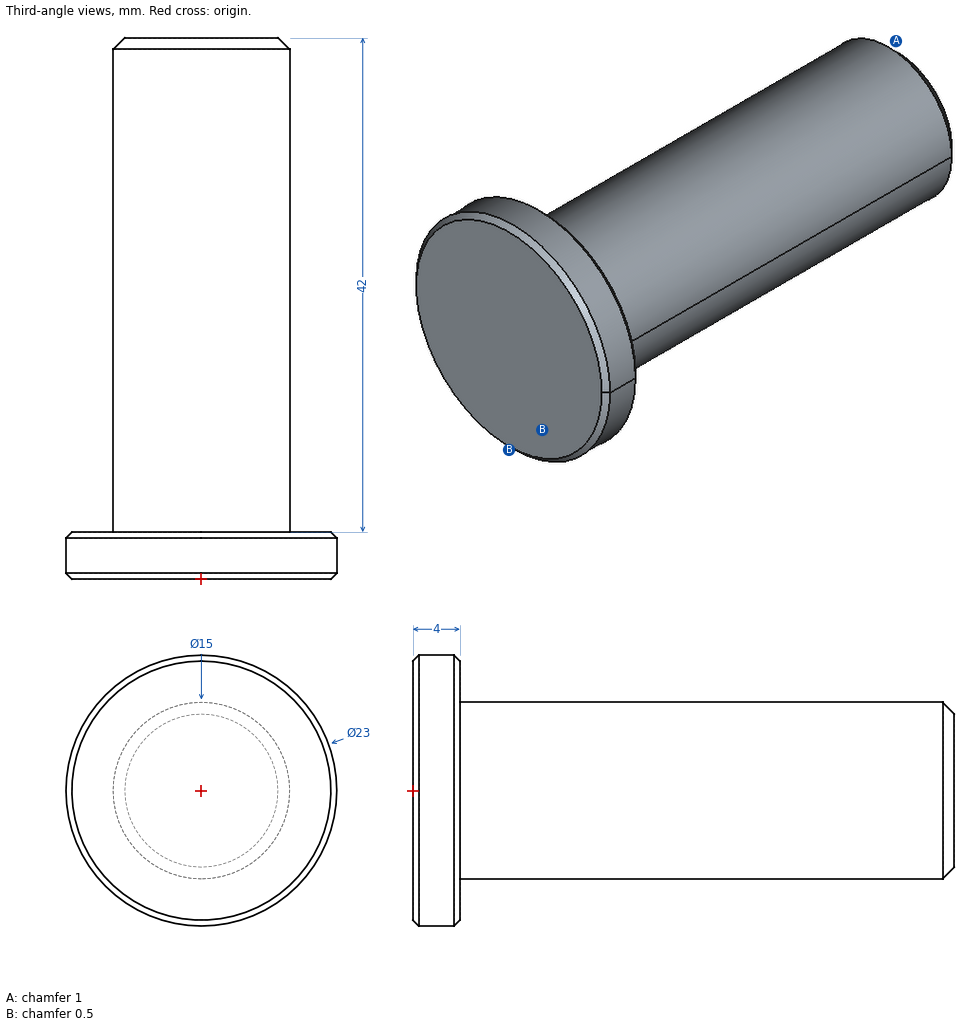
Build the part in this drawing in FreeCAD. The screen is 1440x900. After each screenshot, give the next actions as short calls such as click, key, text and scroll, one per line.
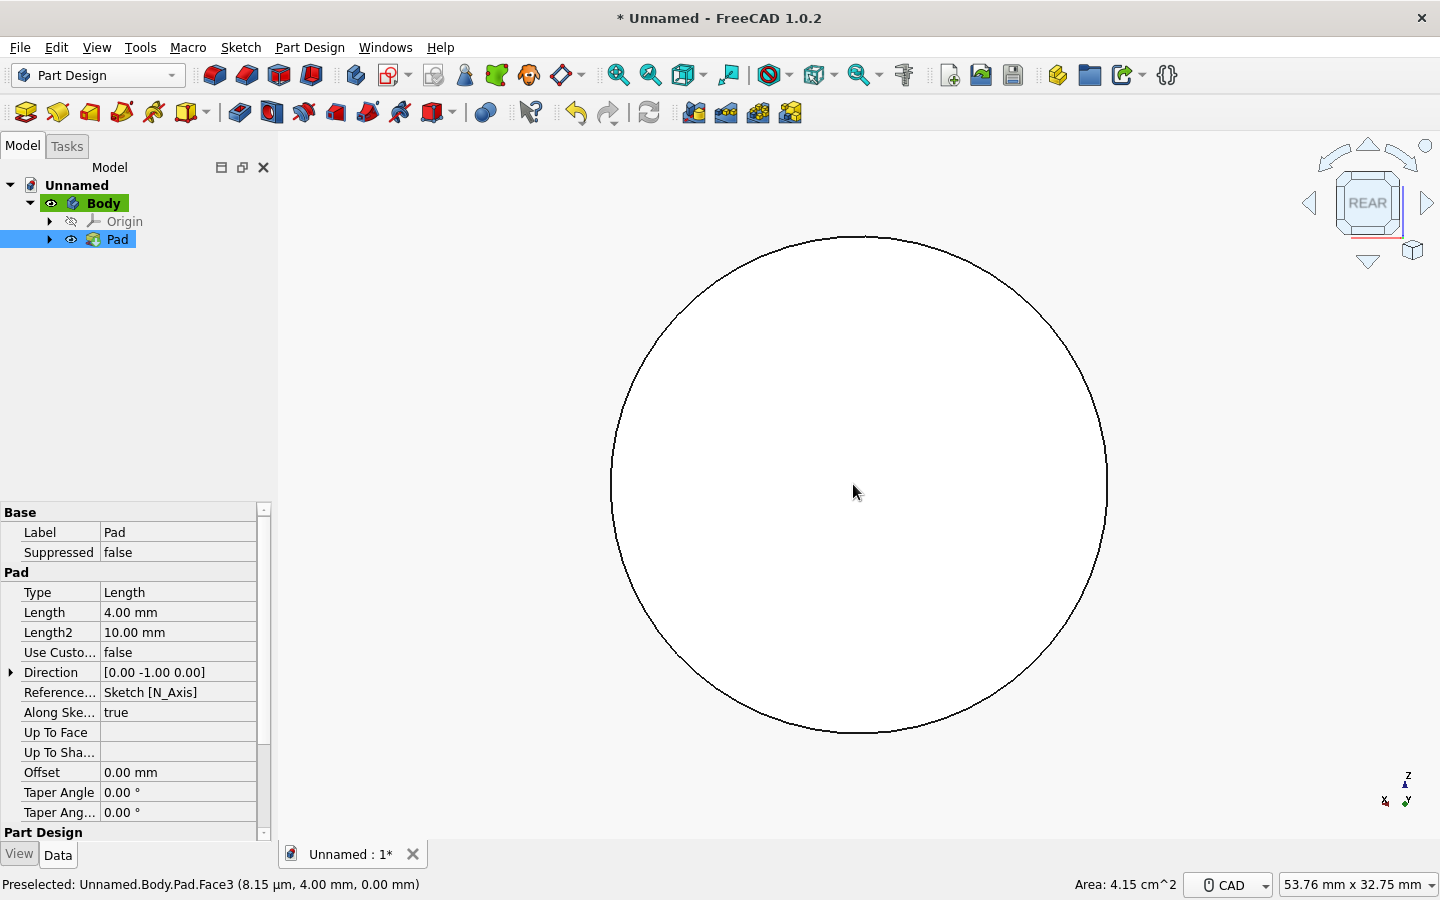
click(388, 76)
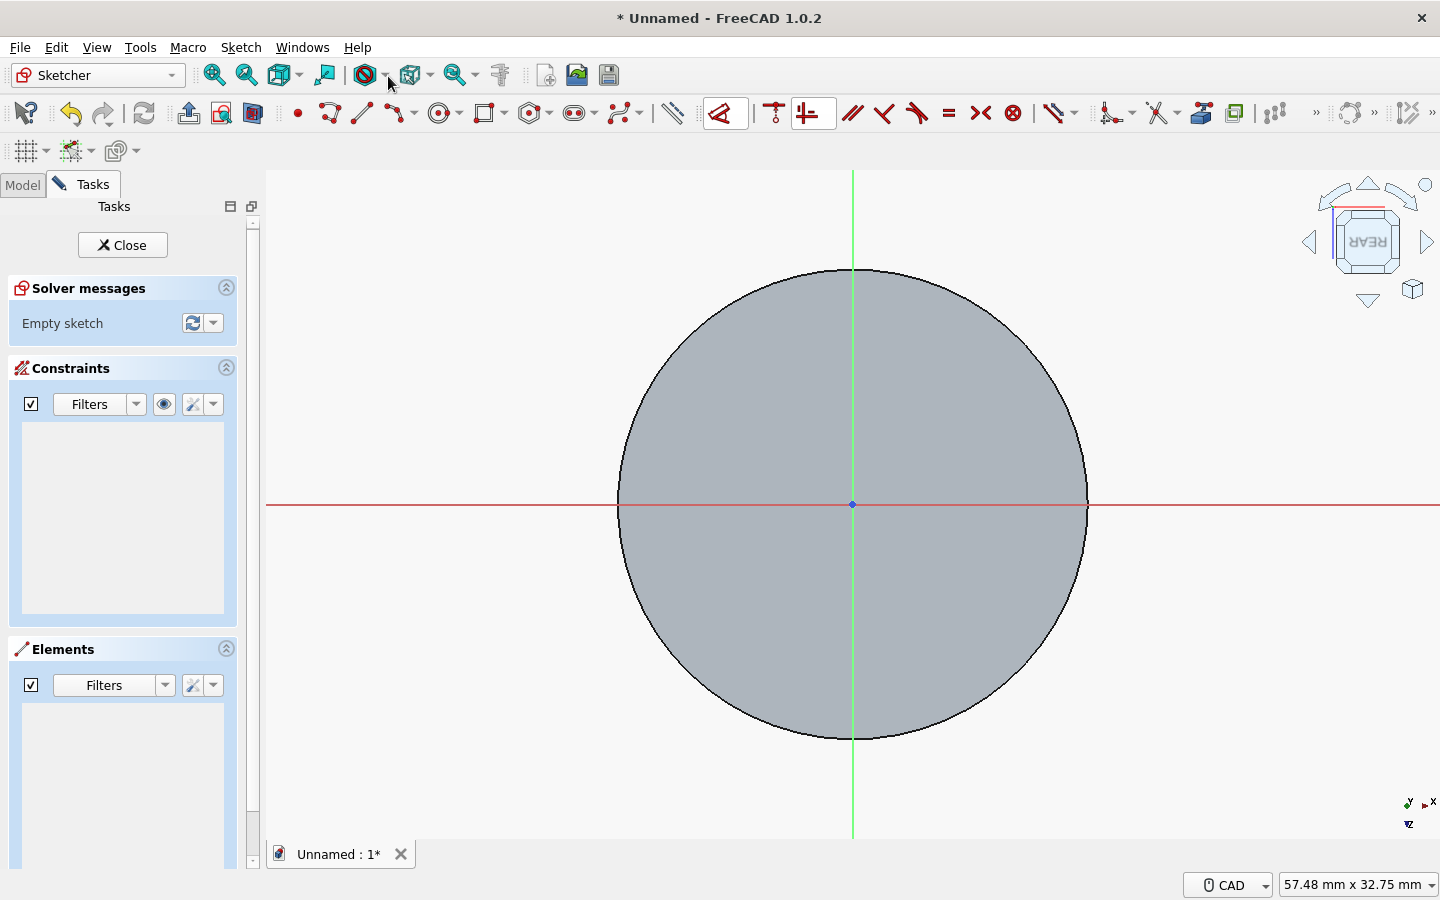
scroll(992, 505, up, 2)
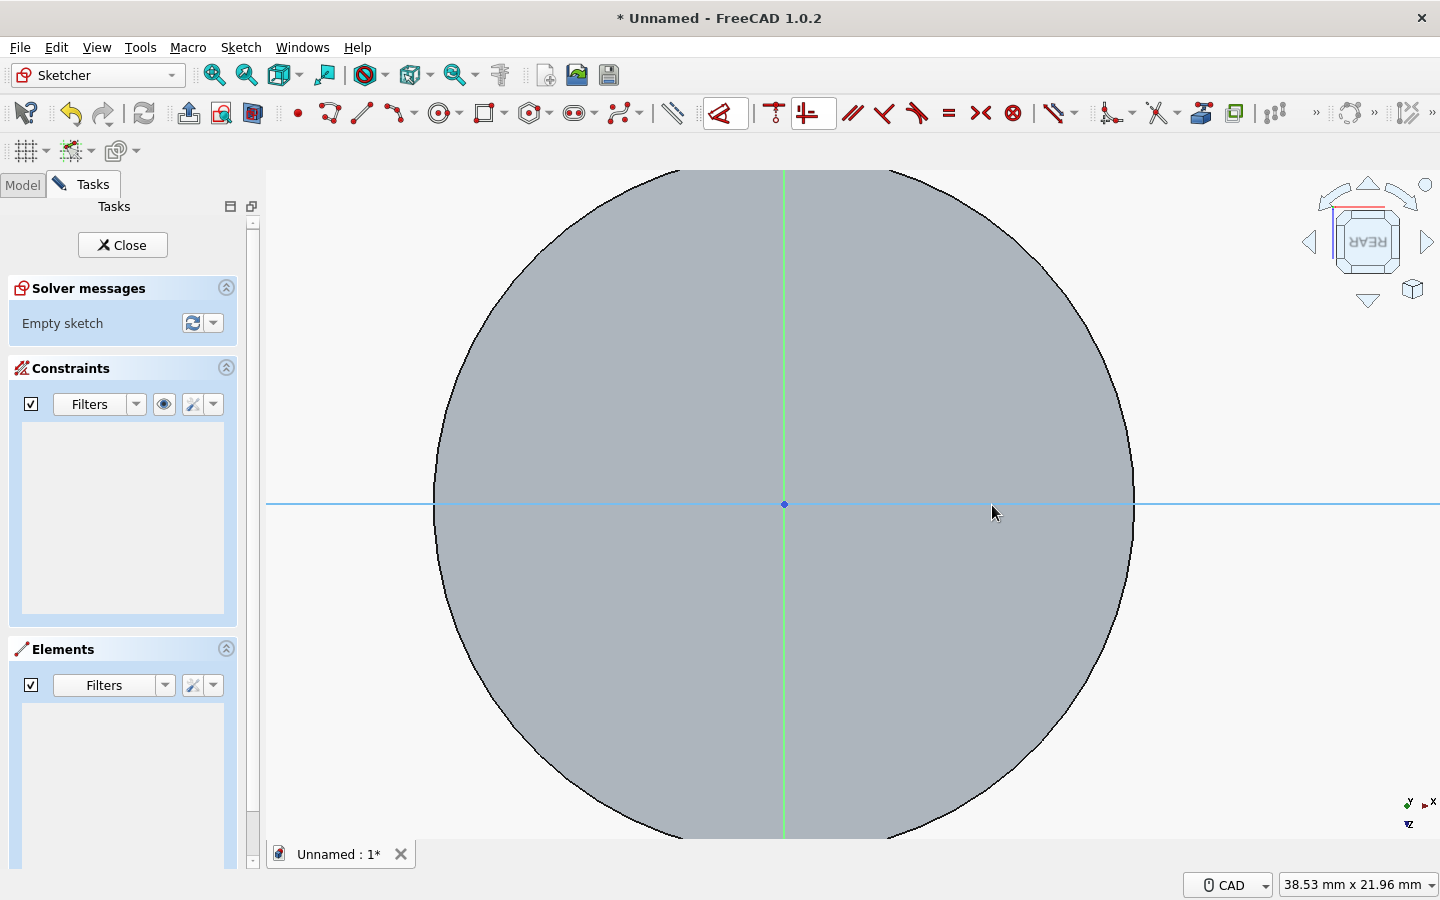
key(g)
key(c)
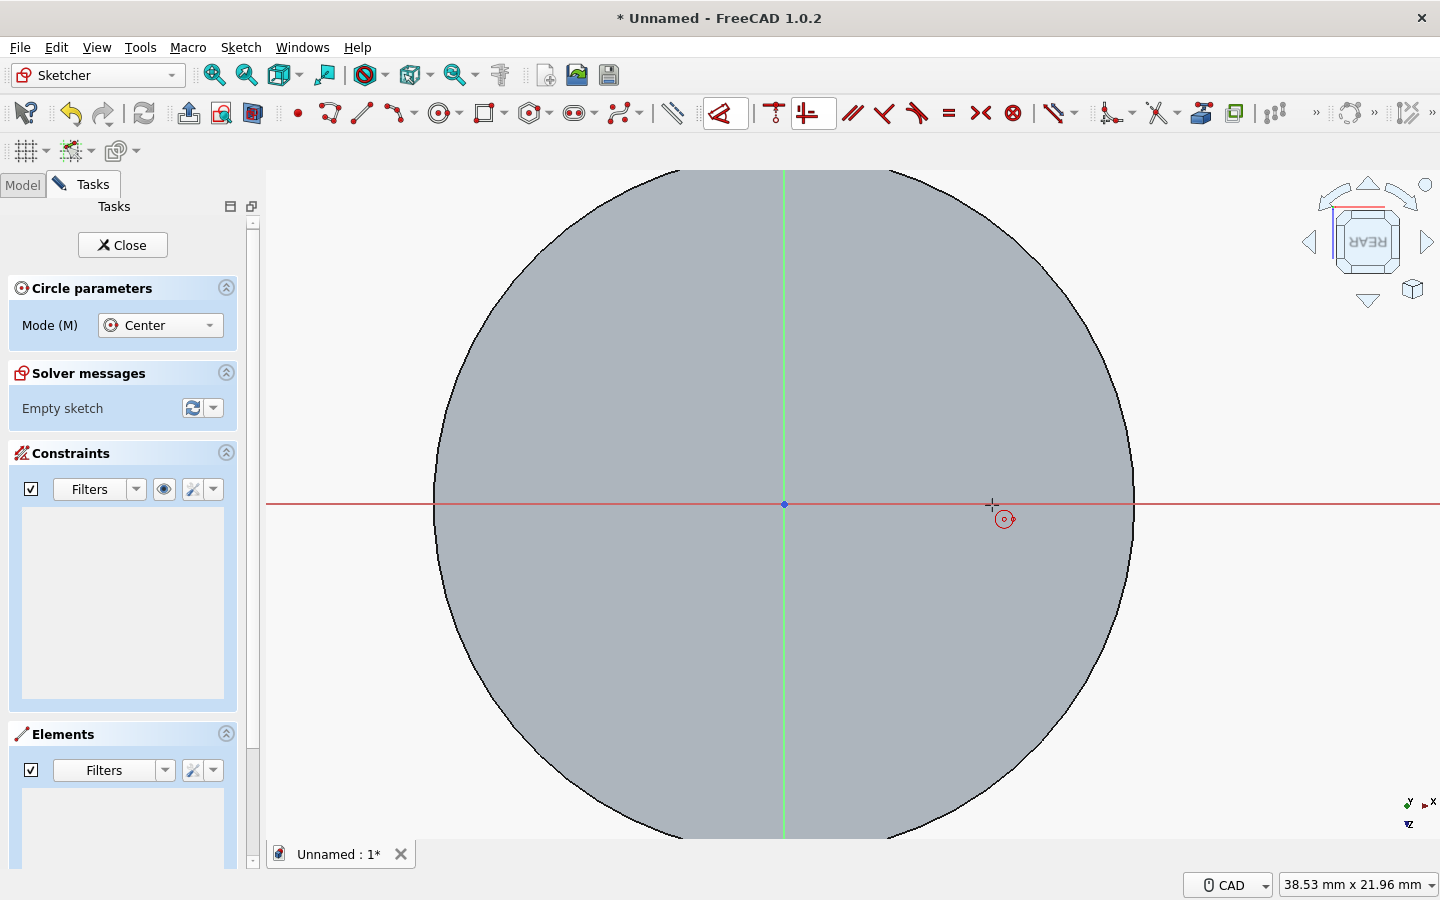
click(784, 504)
move(946, 342)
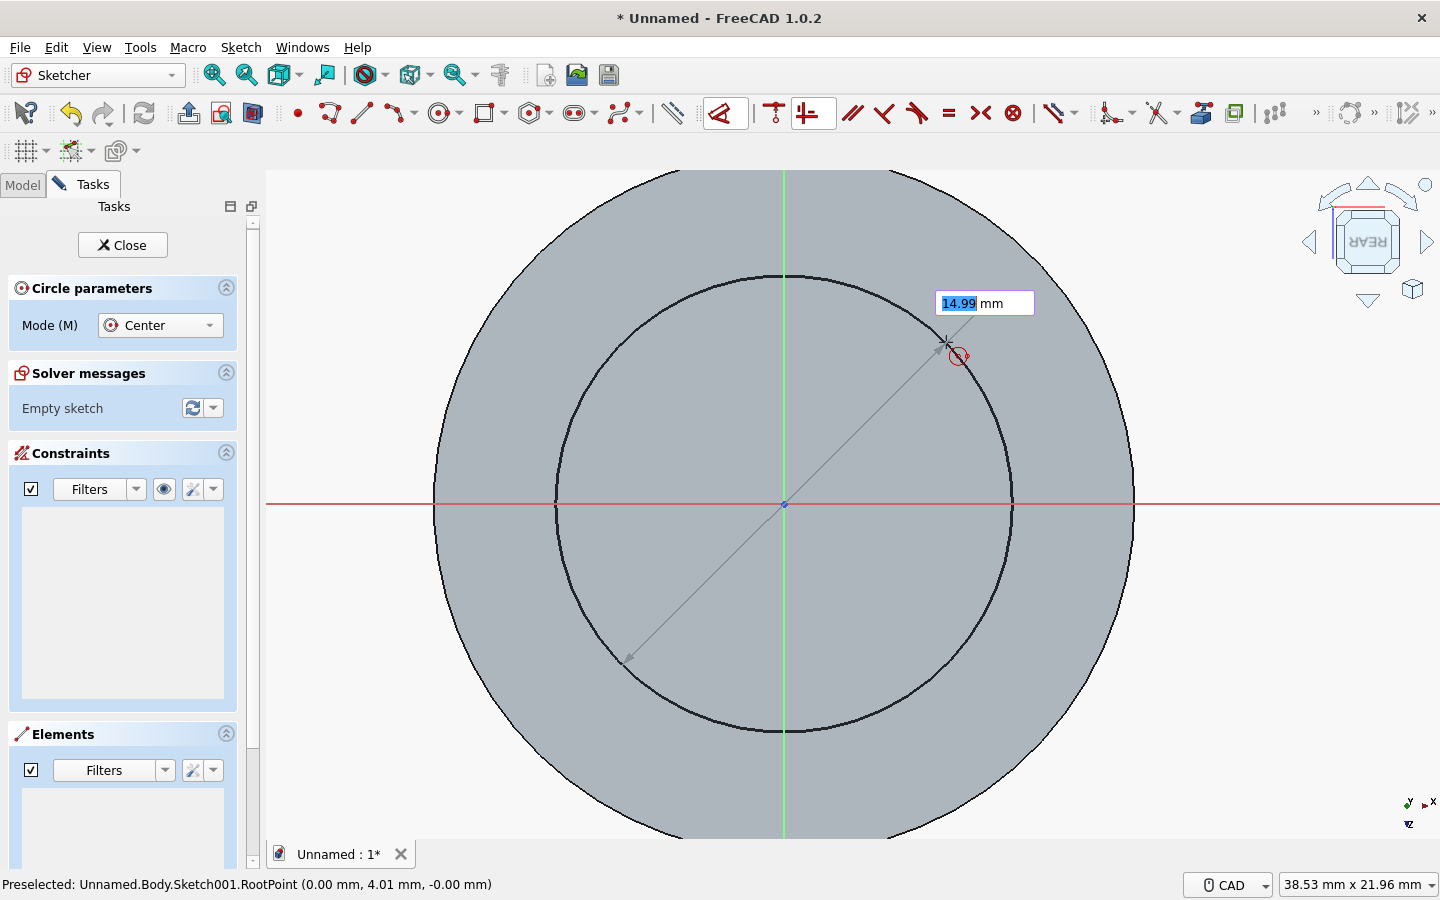
text(15)
key(Return)
key(Escape)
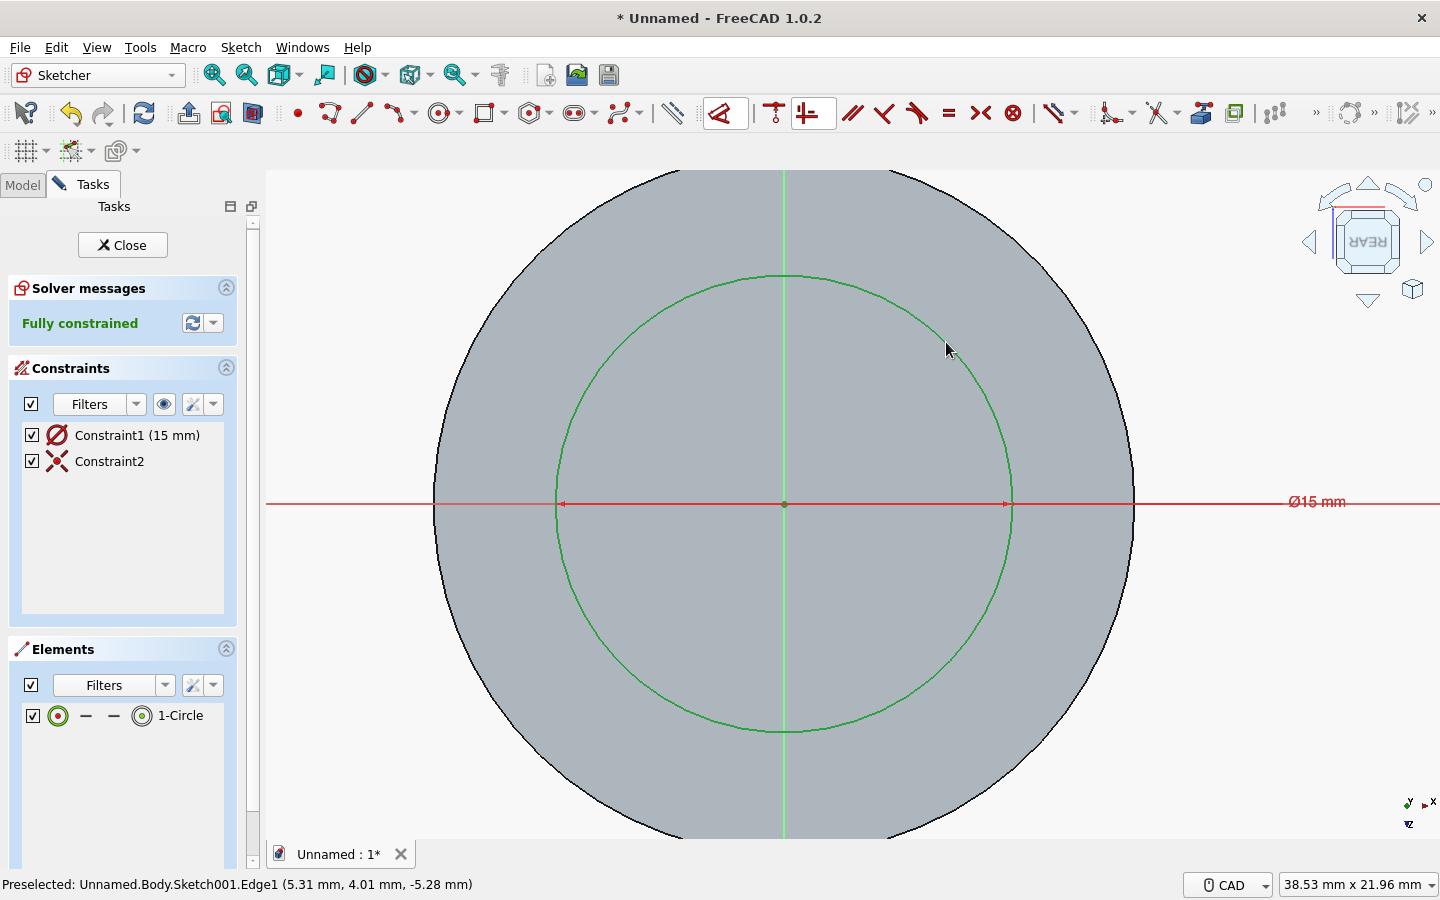
click(123, 245)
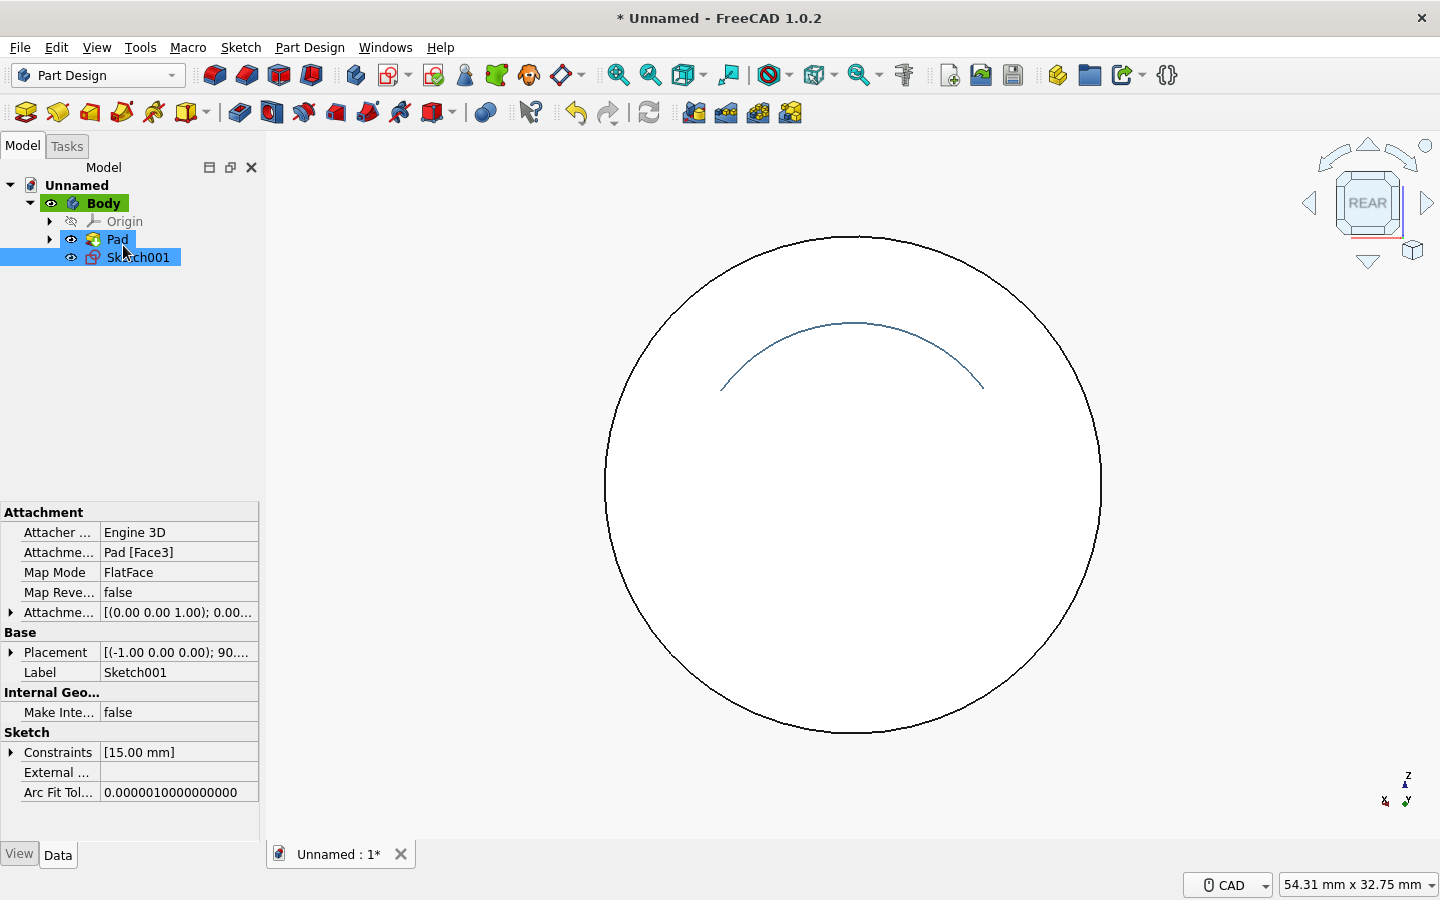
click(26, 112)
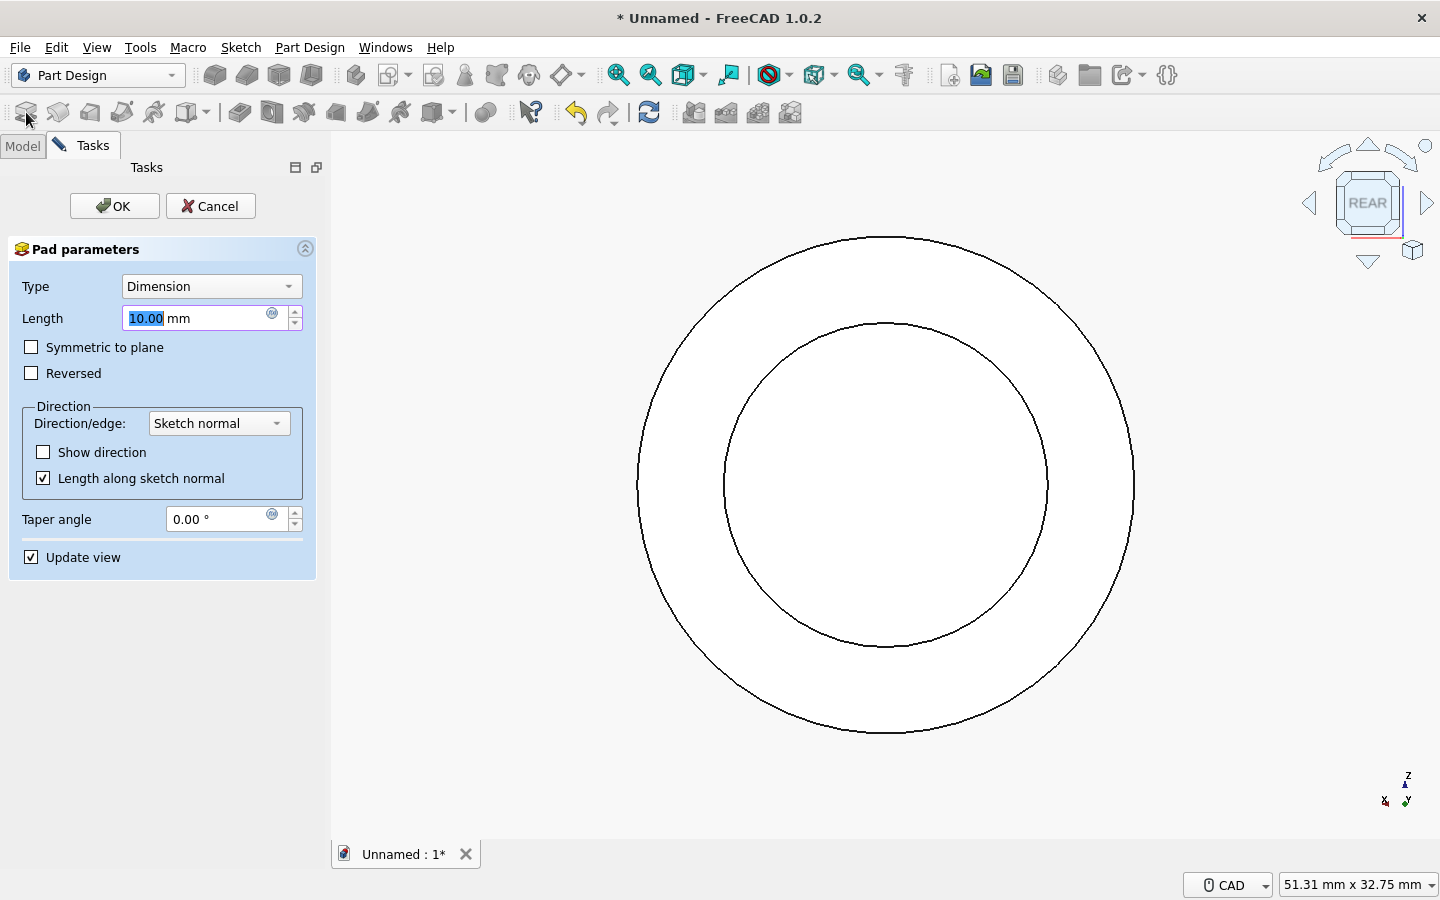
text(42)
key(Tab)